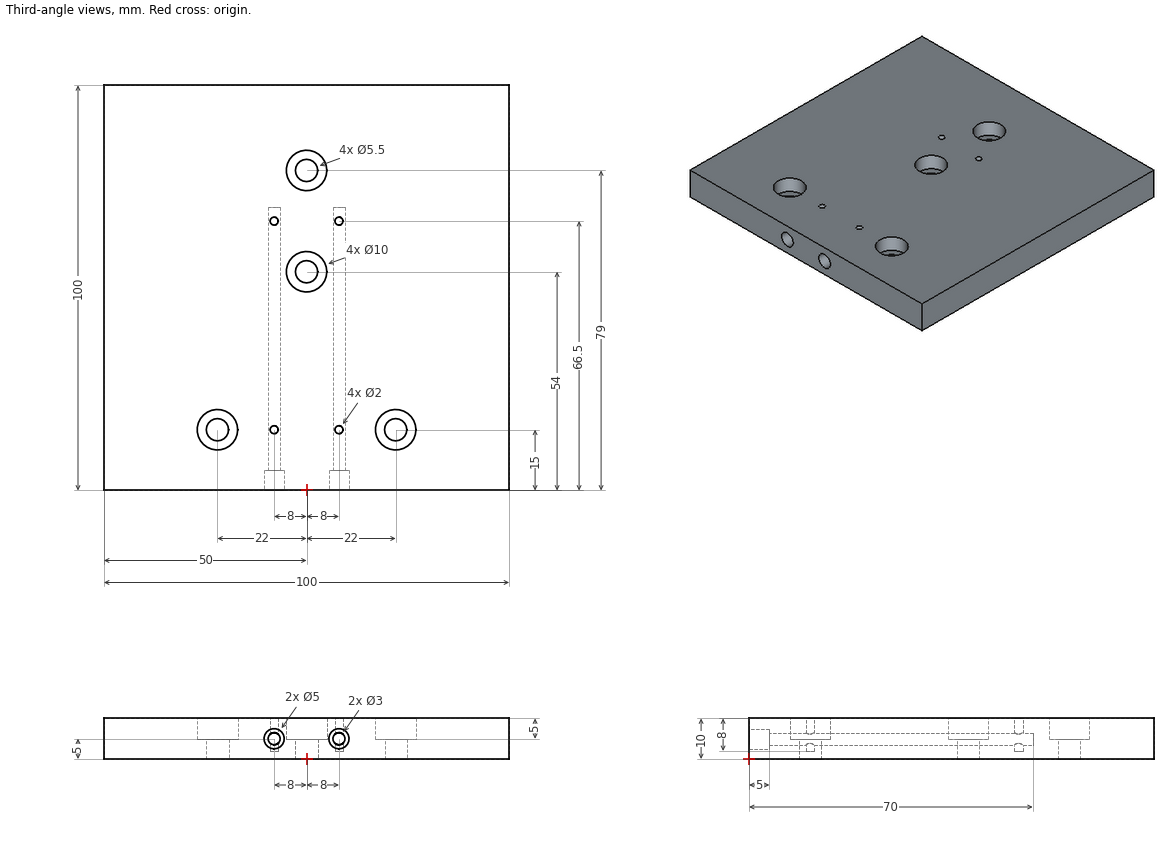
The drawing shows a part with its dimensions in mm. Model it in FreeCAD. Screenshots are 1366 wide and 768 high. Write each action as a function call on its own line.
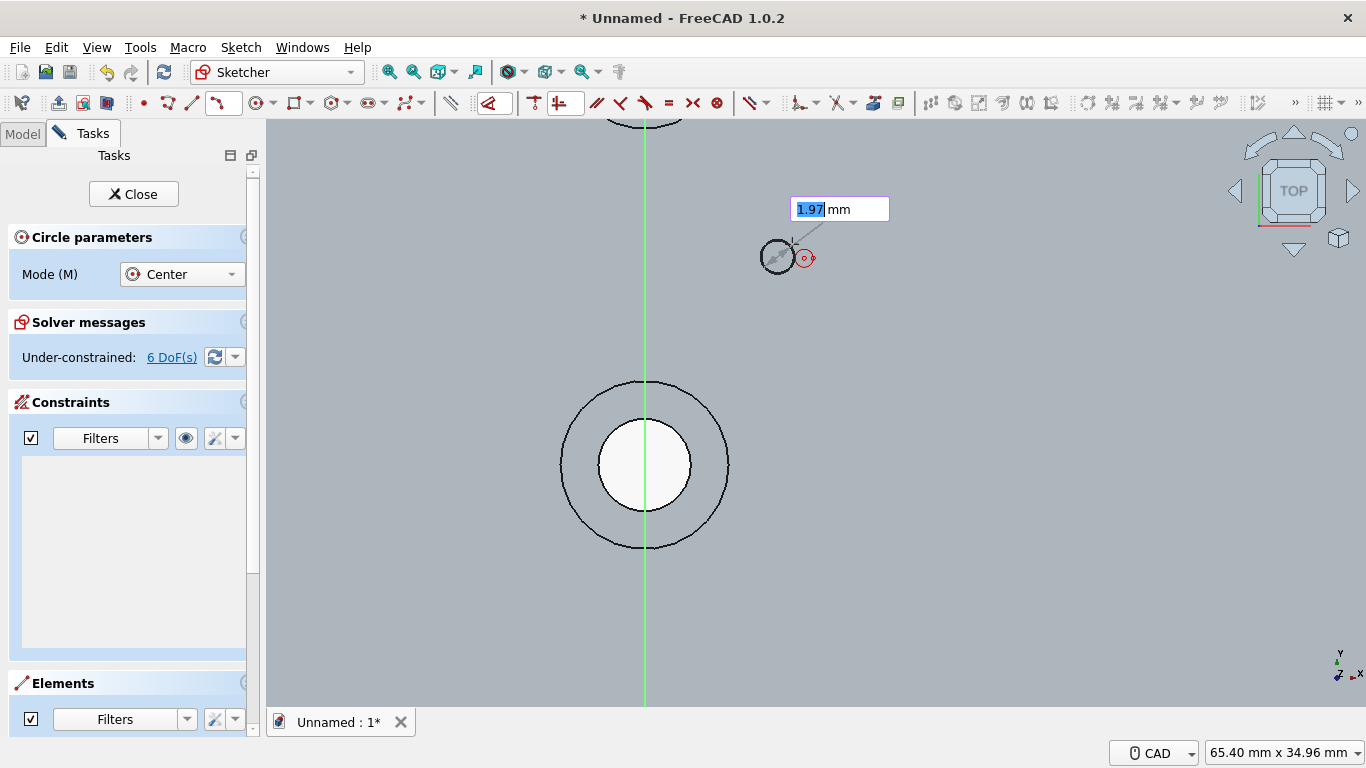
click(791, 243)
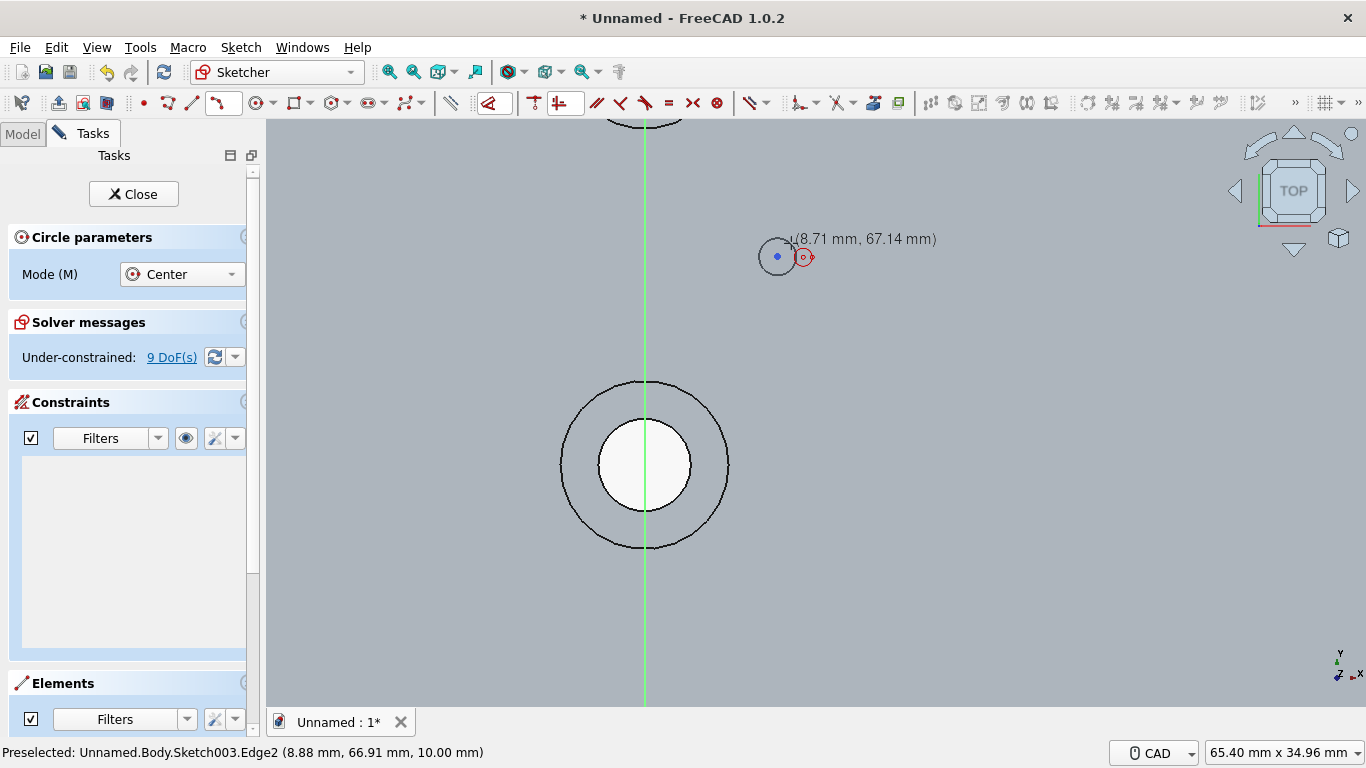
scroll(510, 255, up, 2)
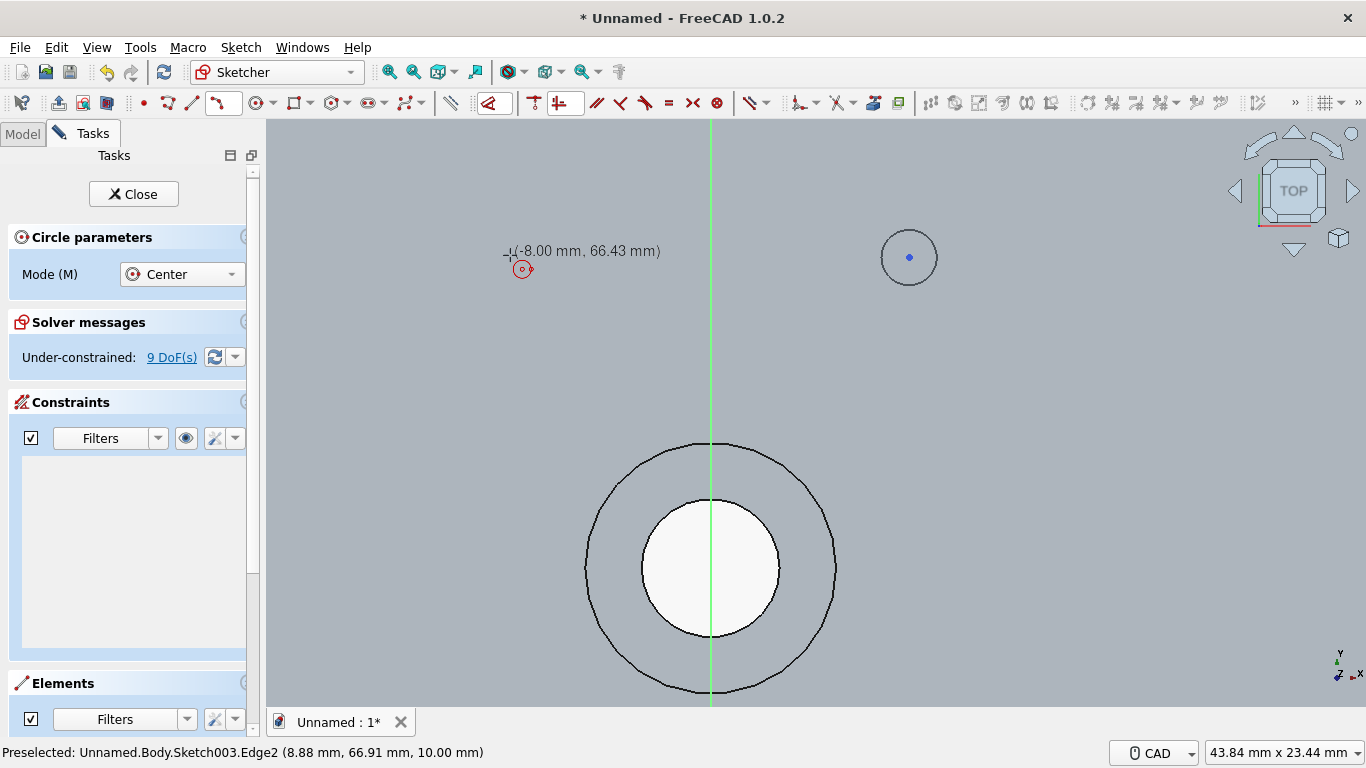
scroll(757, 245, down, 8)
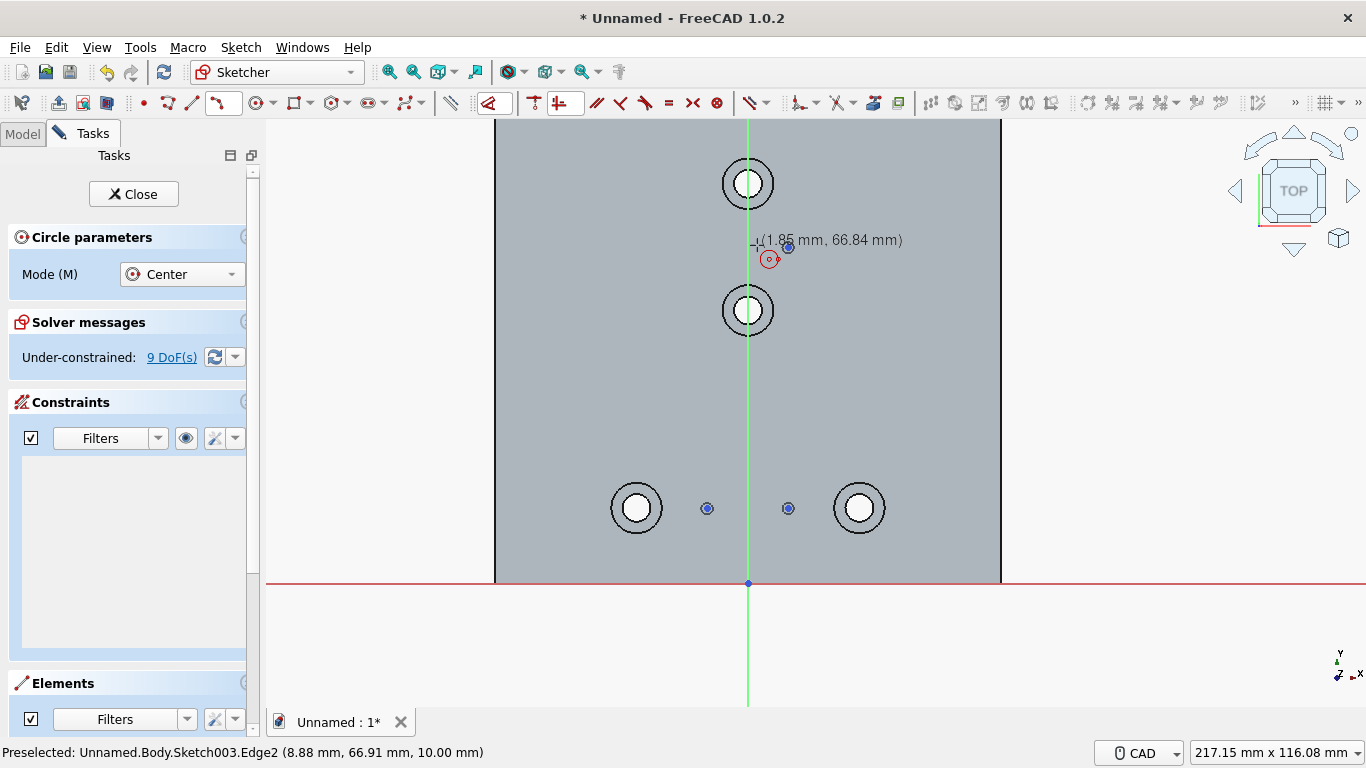
click(707, 247)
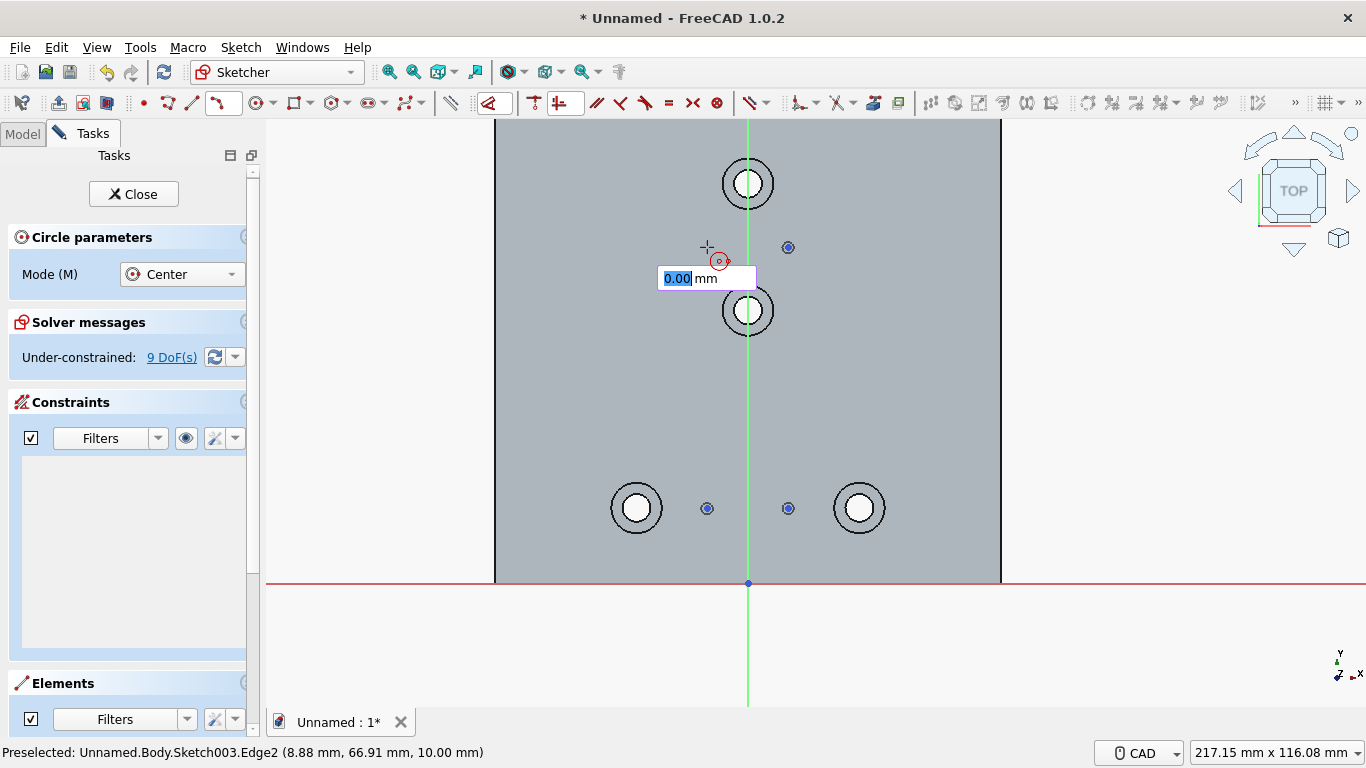
scroll(711, 244, up, 6)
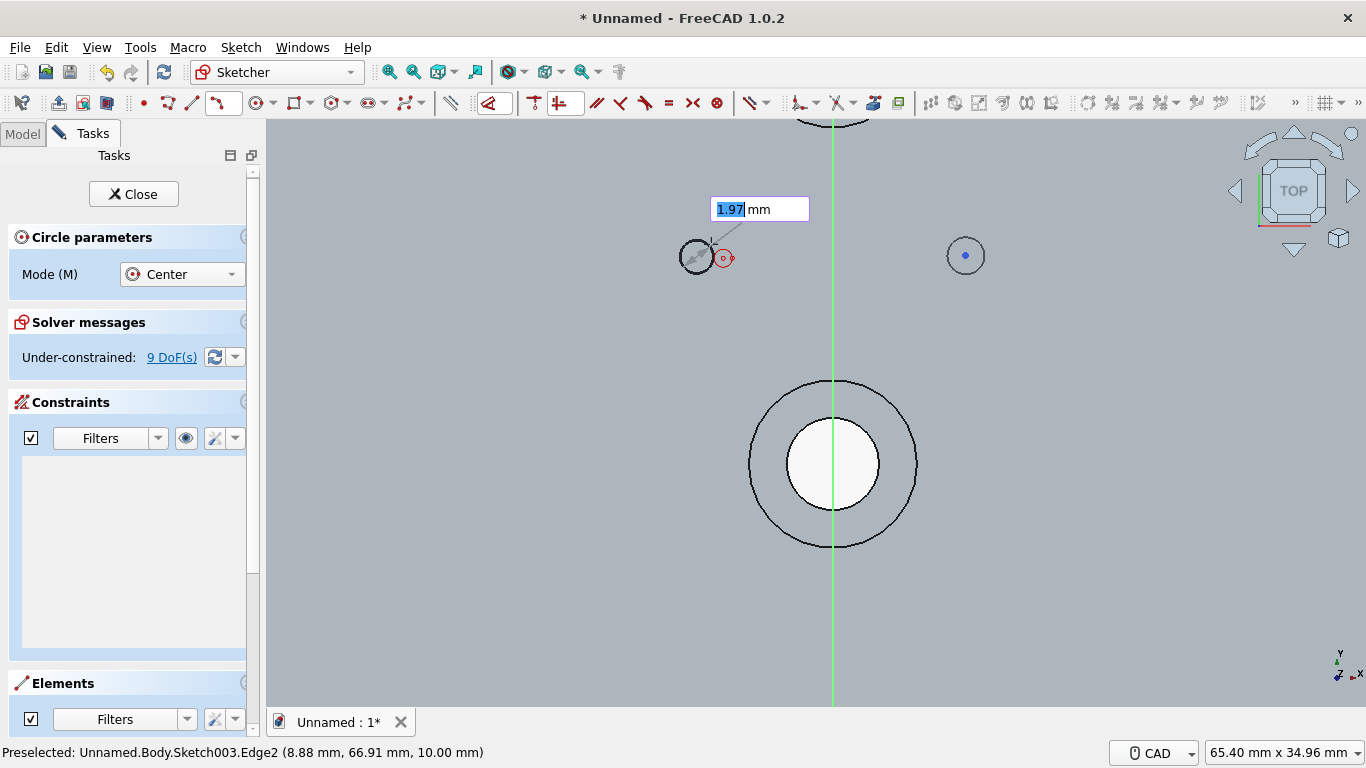
click(710, 242)
key(Escape)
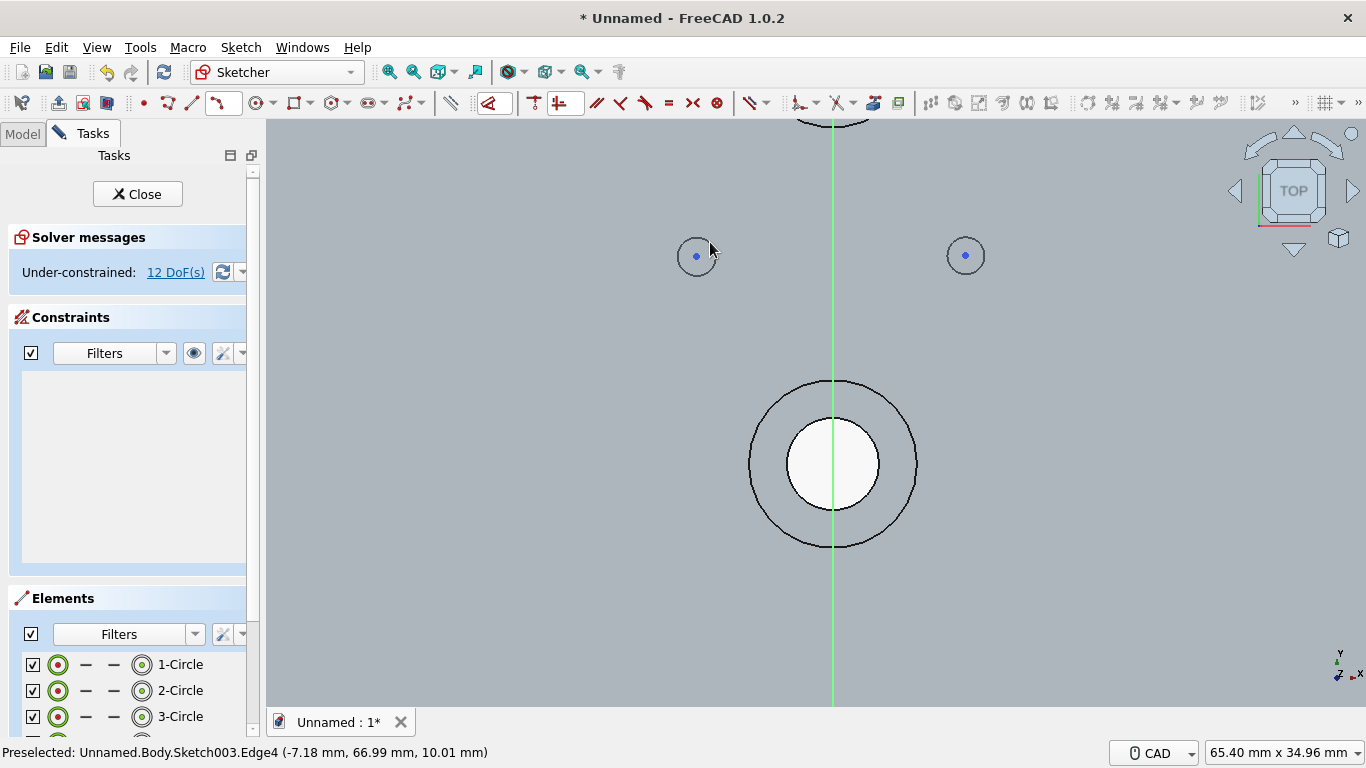
scroll(711, 244, down, 6)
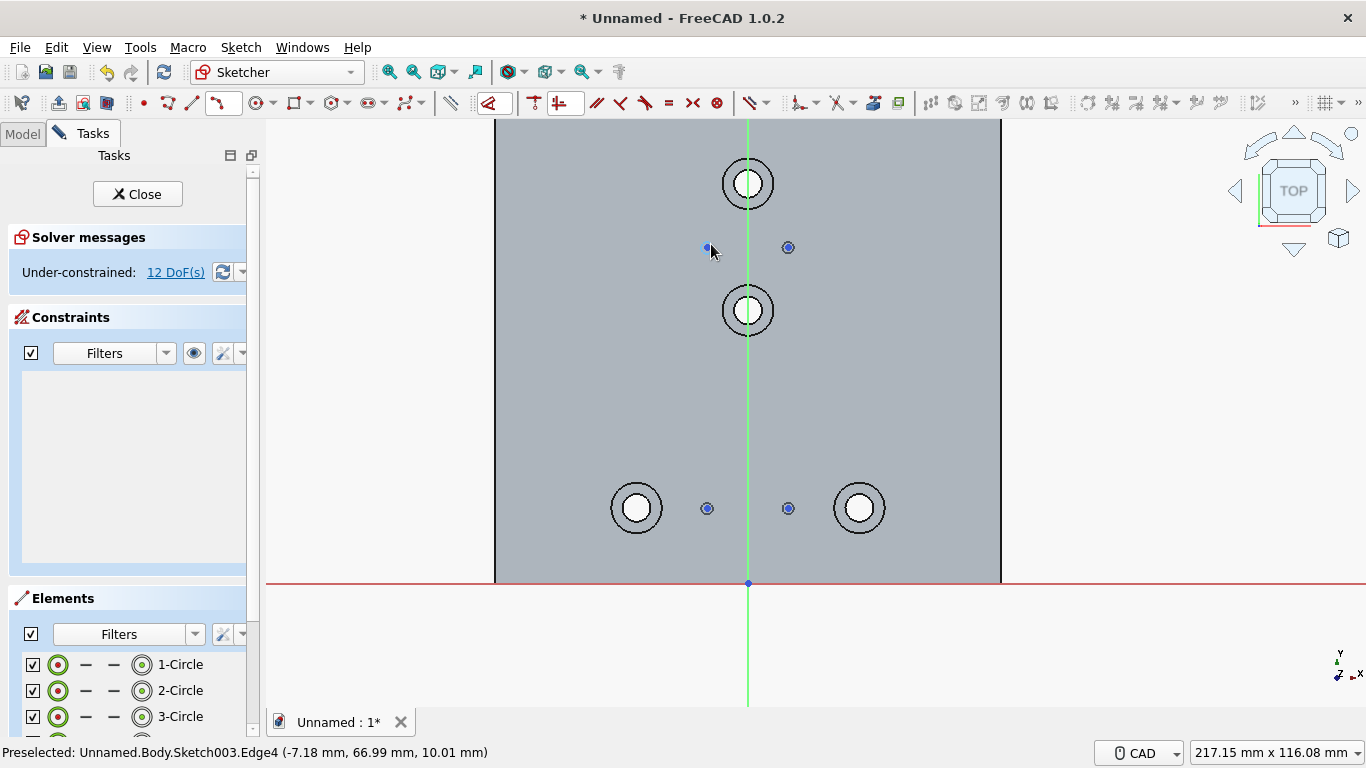
scroll(792, 505, up, 5)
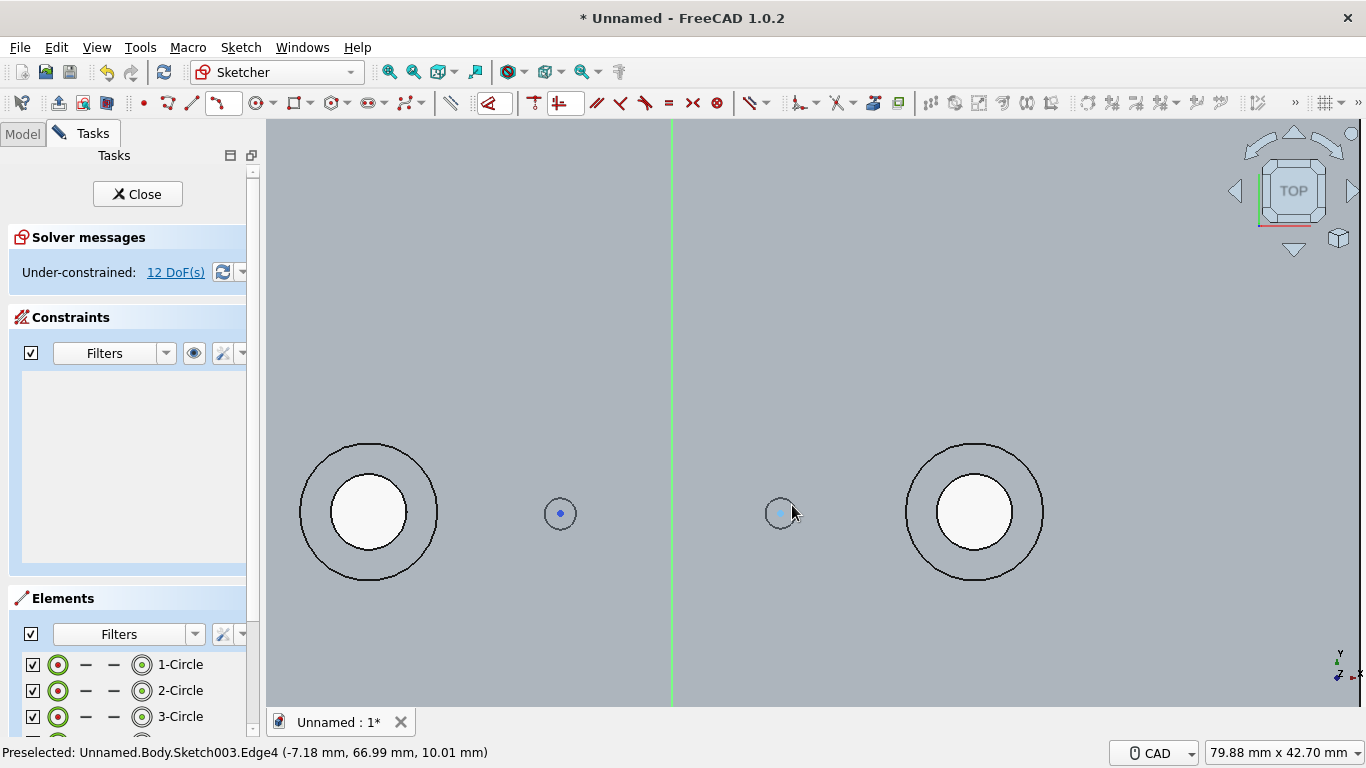
click(791, 503)